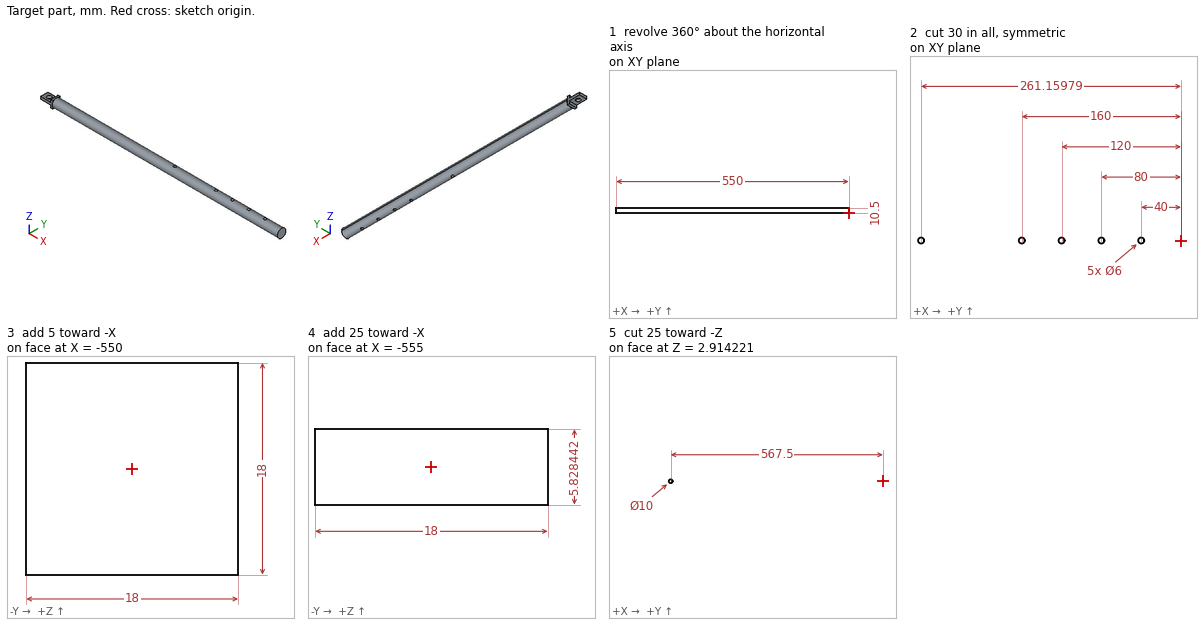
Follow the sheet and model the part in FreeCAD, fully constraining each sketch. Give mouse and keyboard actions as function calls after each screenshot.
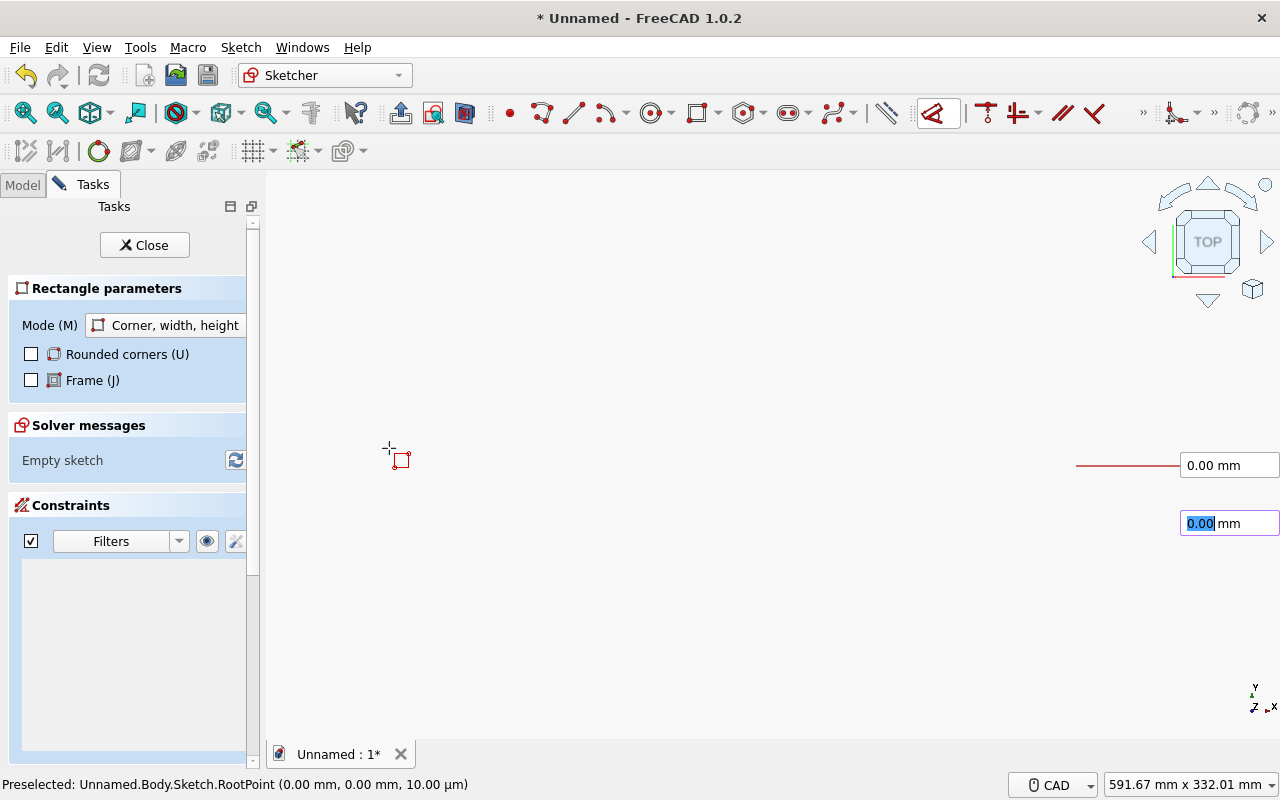
click(389, 448)
key(Escape)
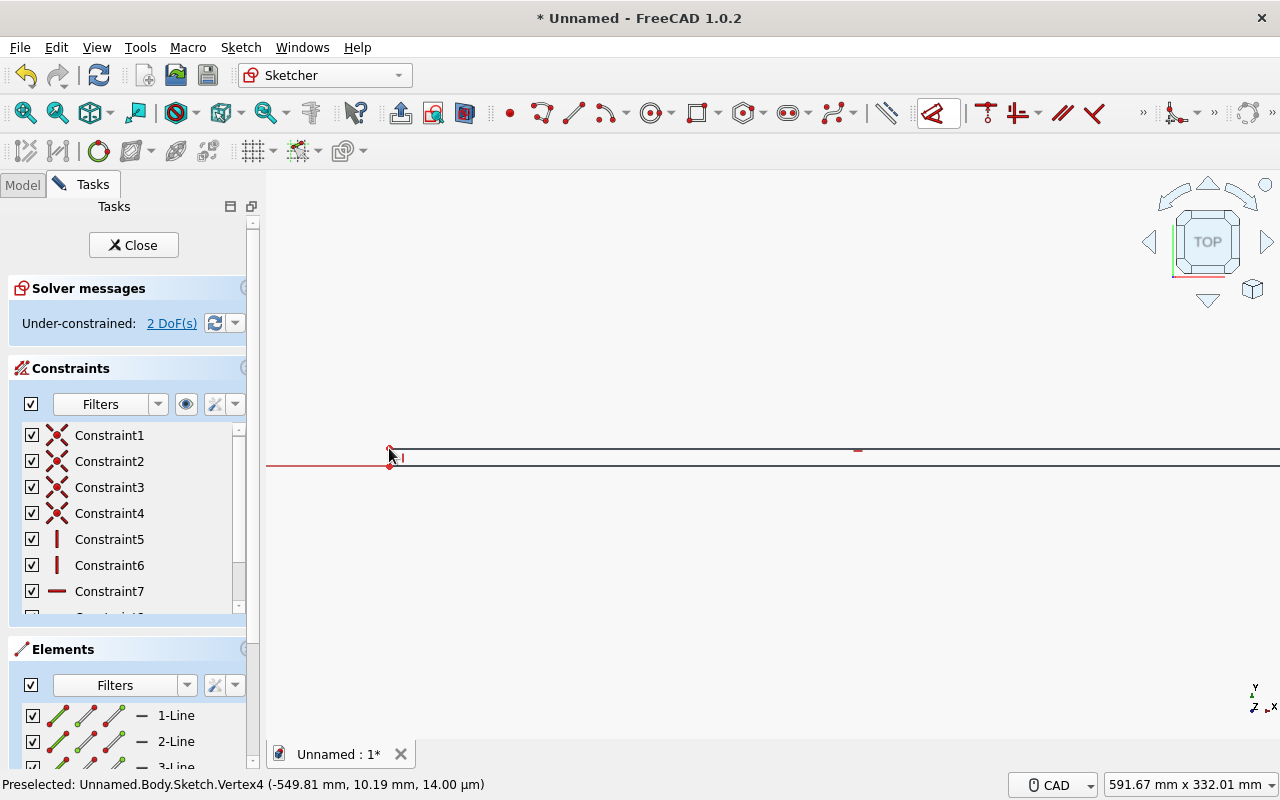
key(d)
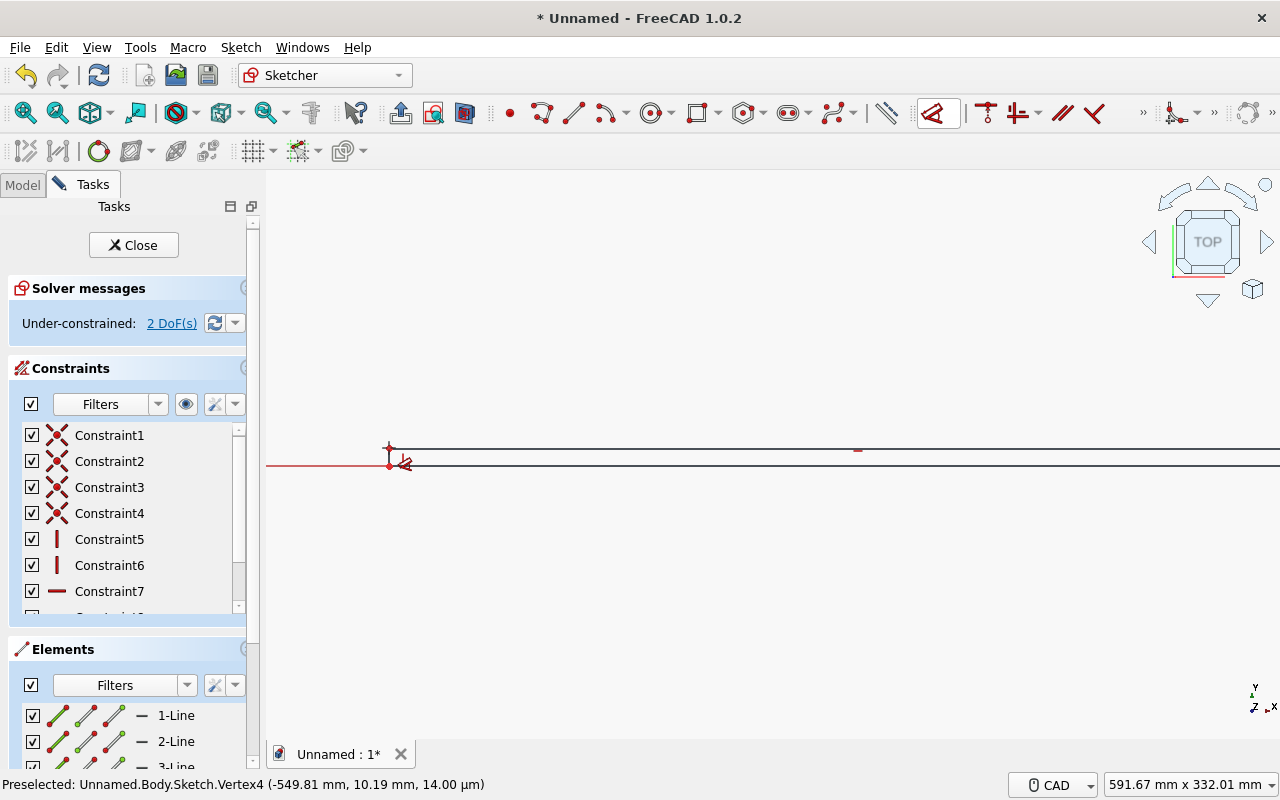
click(1049, 449)
click(752, 415)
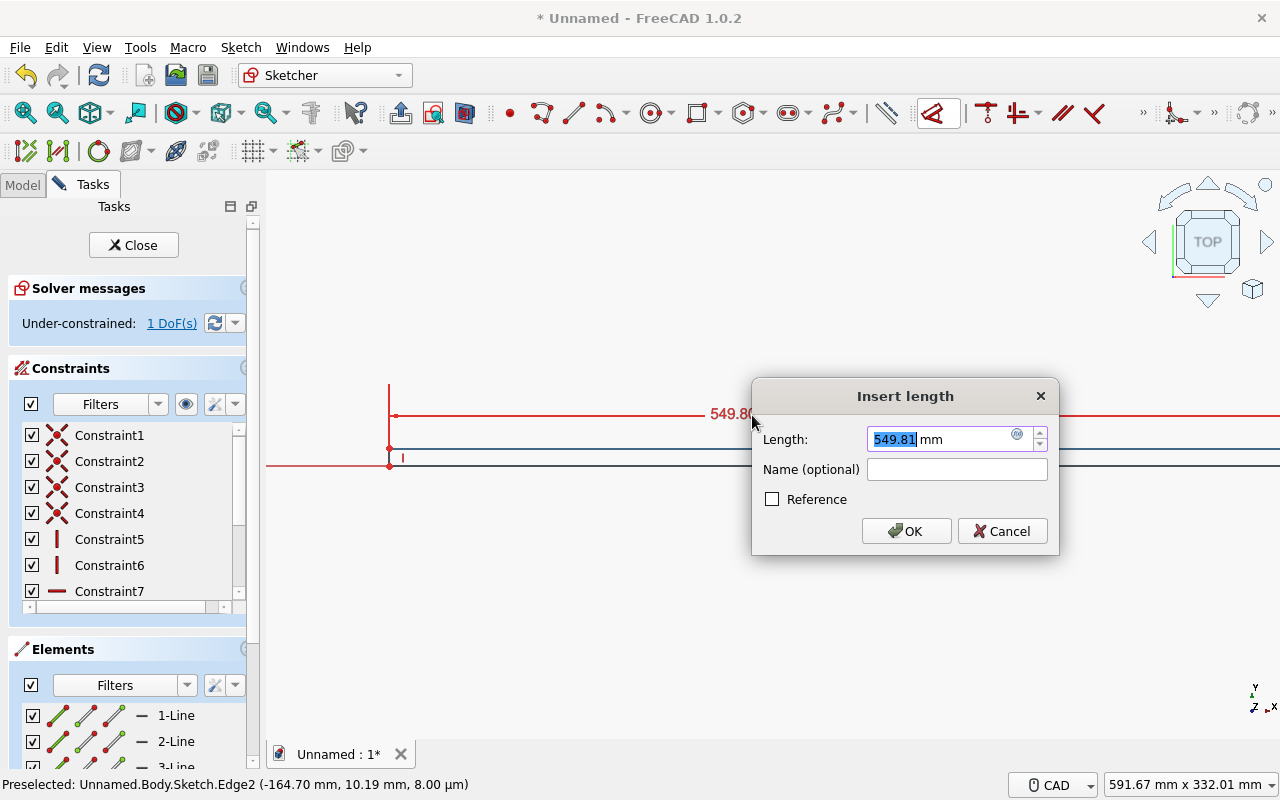
text(550)
key(Return)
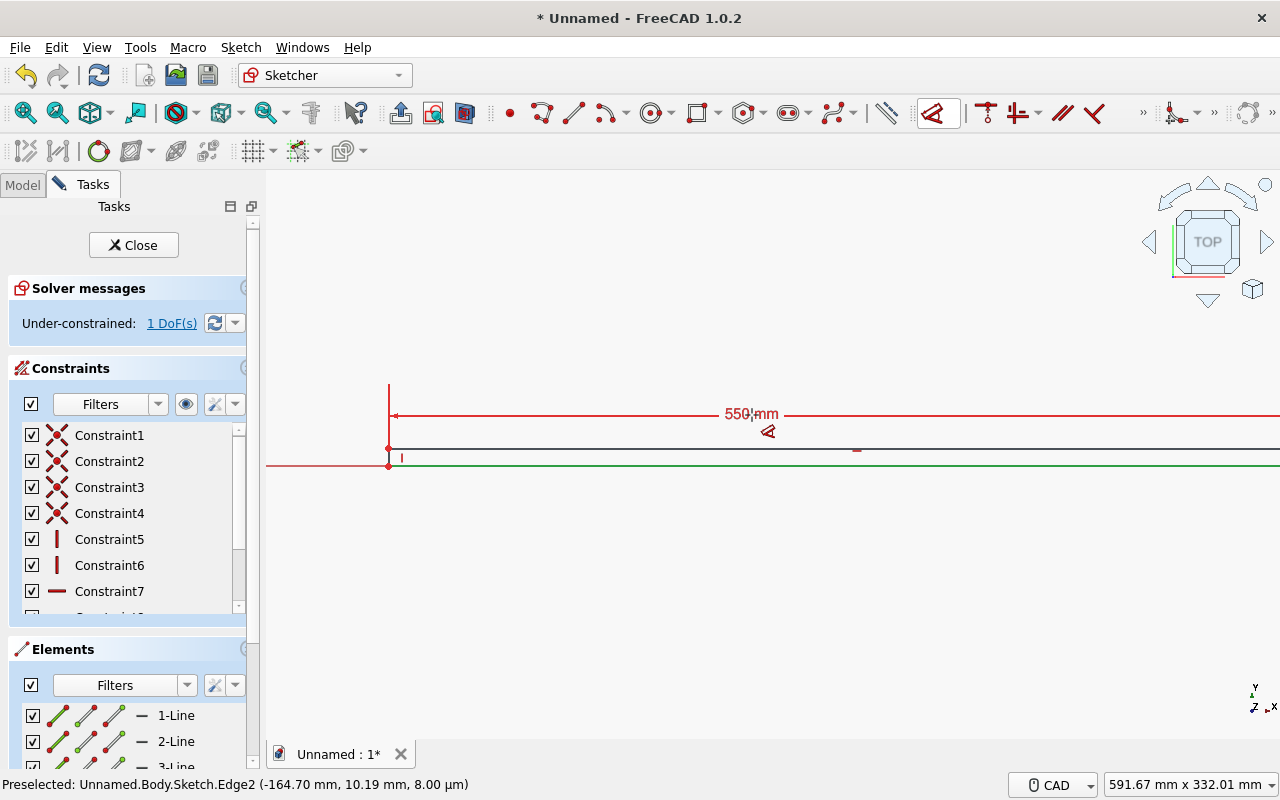
scroll(388, 448, down, 2)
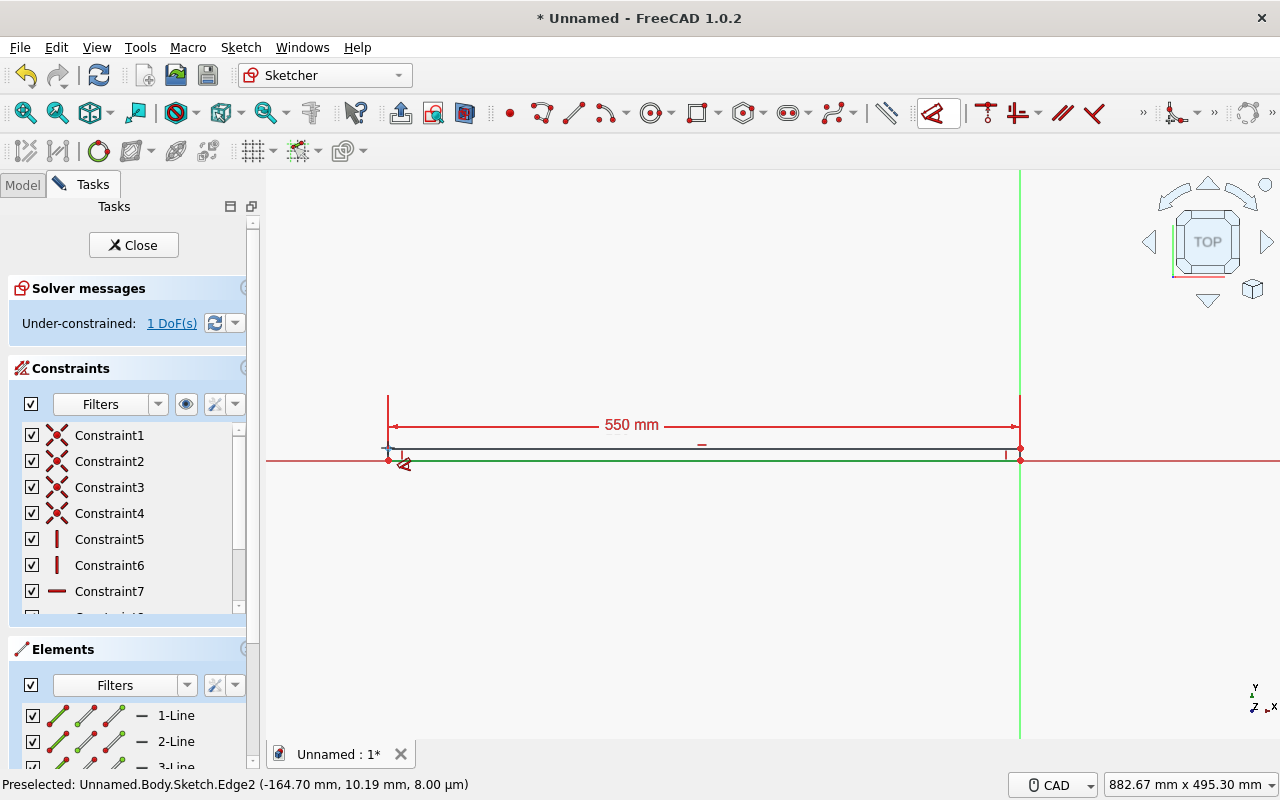
scroll(1020, 455, up, 6)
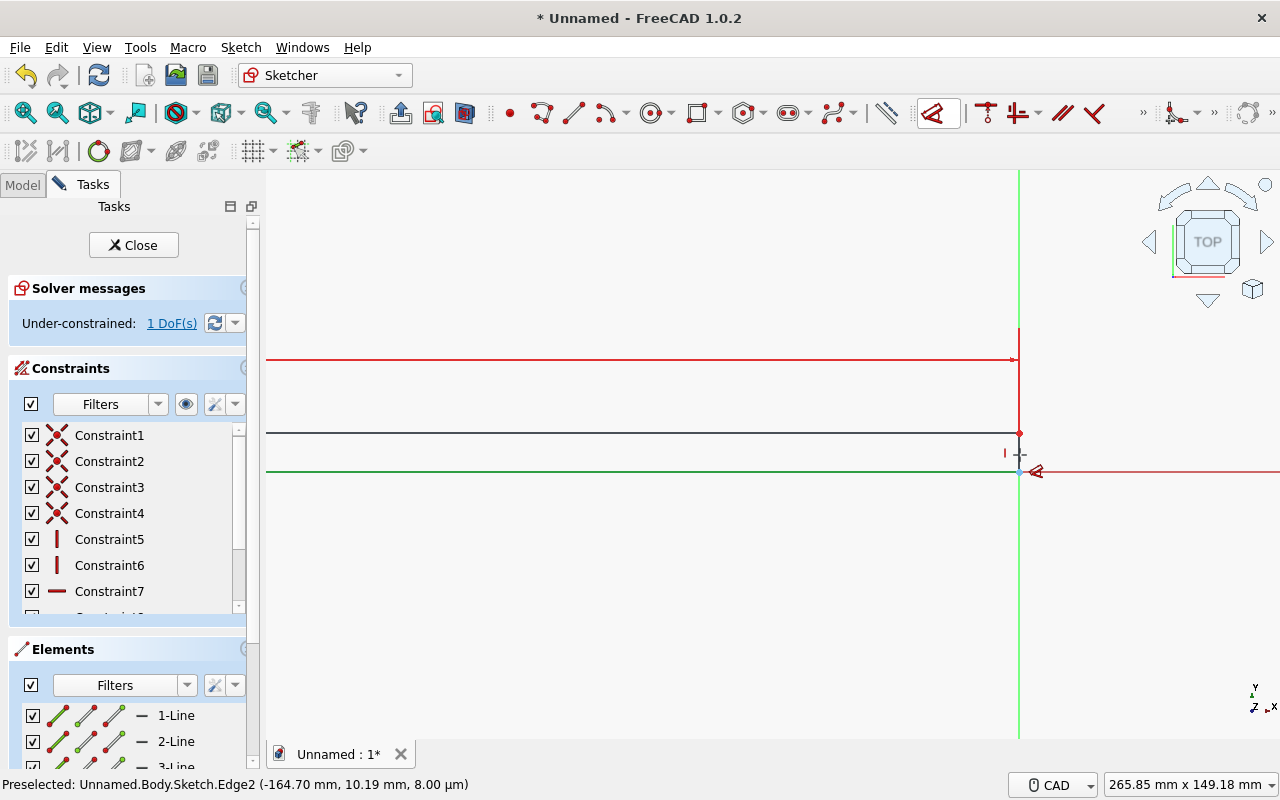
click(1019, 453)
click(1053, 453)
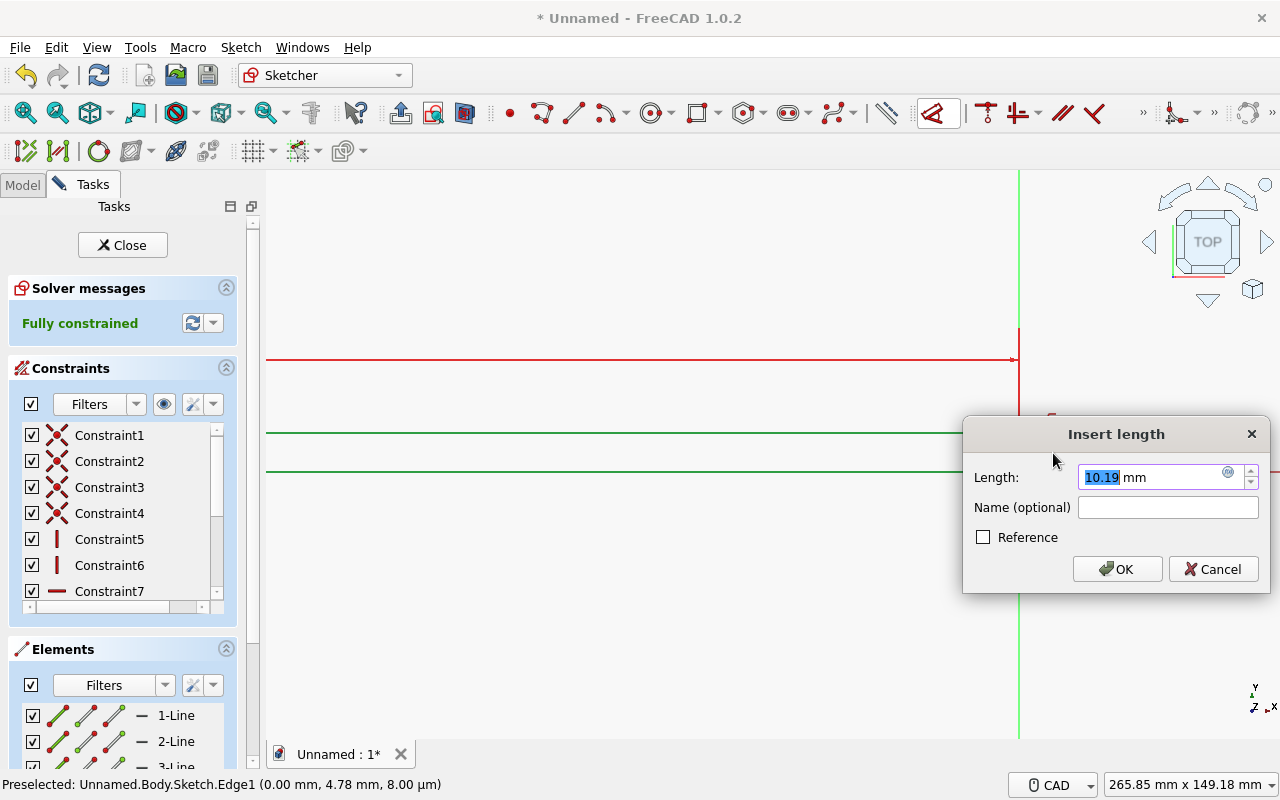
text(10.5)
key(Return)
key(Escape)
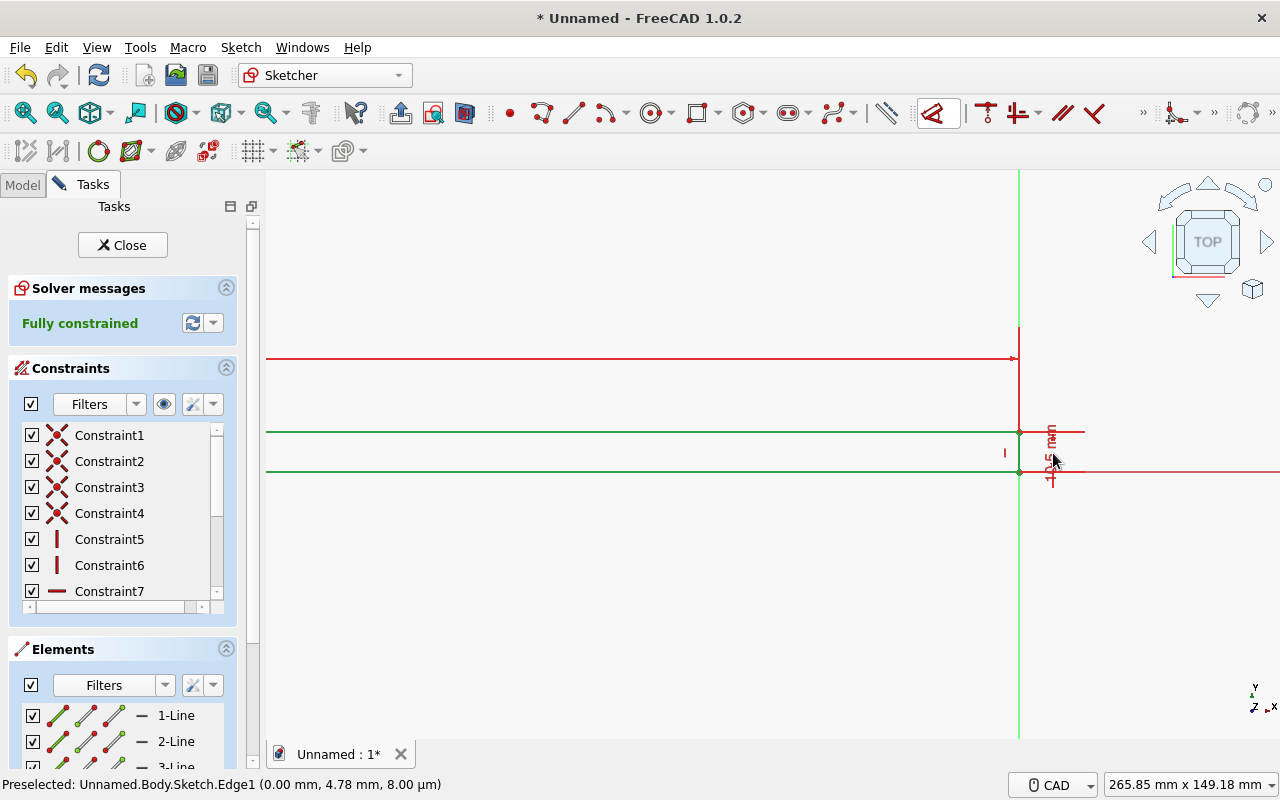
click(123, 245)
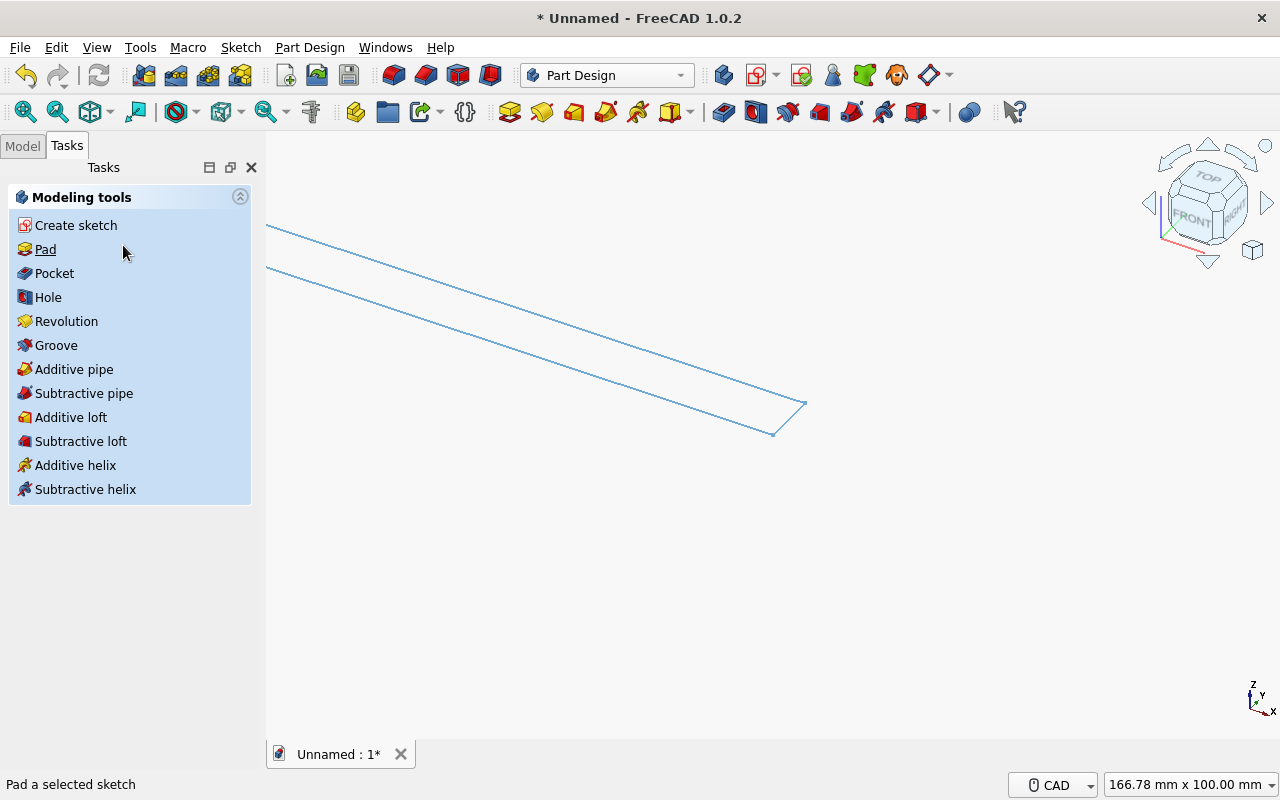
click(542, 112)